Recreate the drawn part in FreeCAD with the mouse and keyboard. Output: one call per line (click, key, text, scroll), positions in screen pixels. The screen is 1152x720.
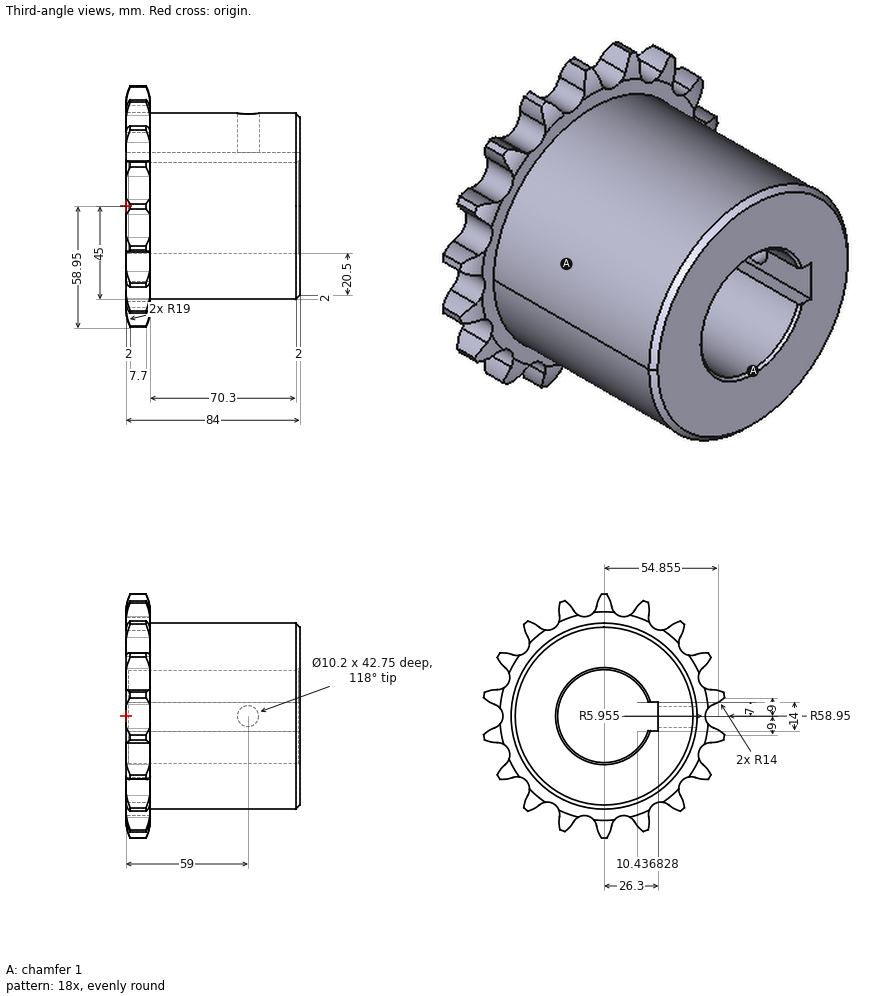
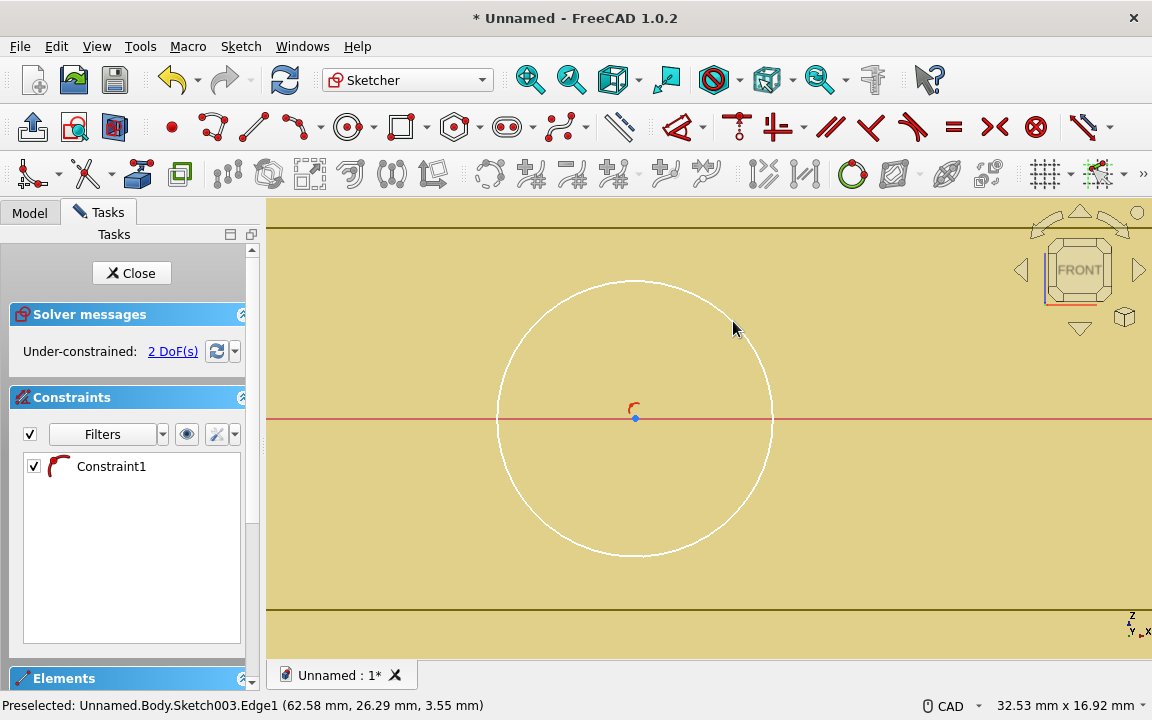
click(676, 128)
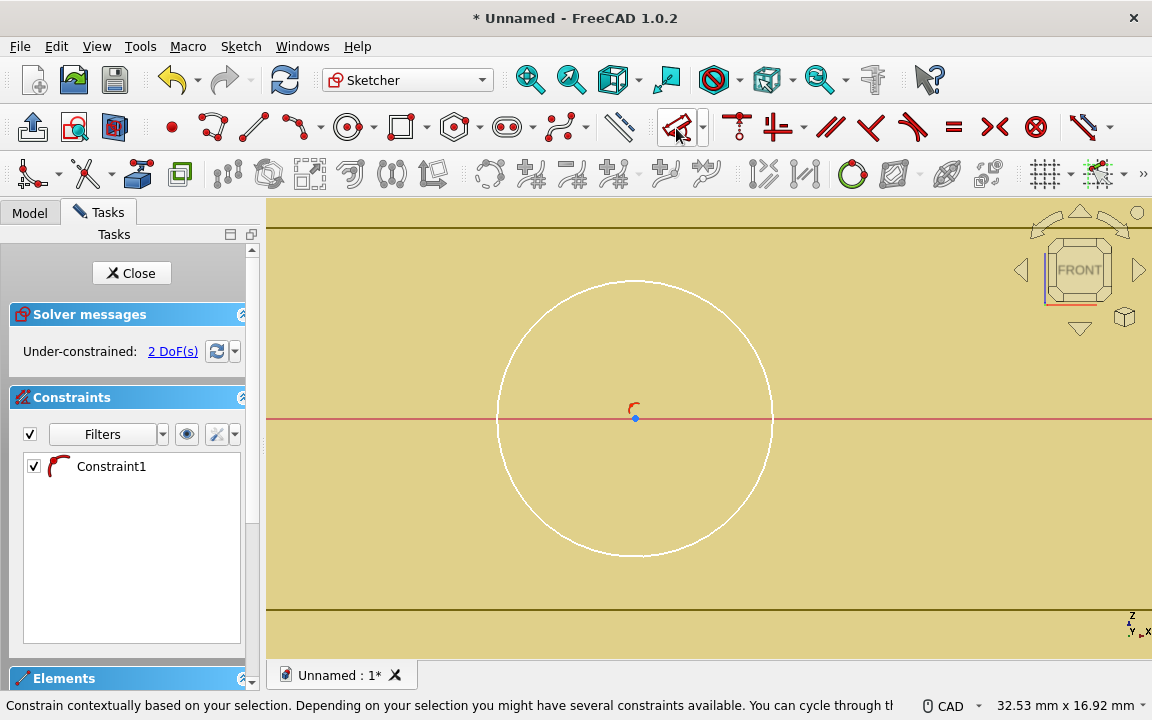
click(732, 321)
click(755, 298)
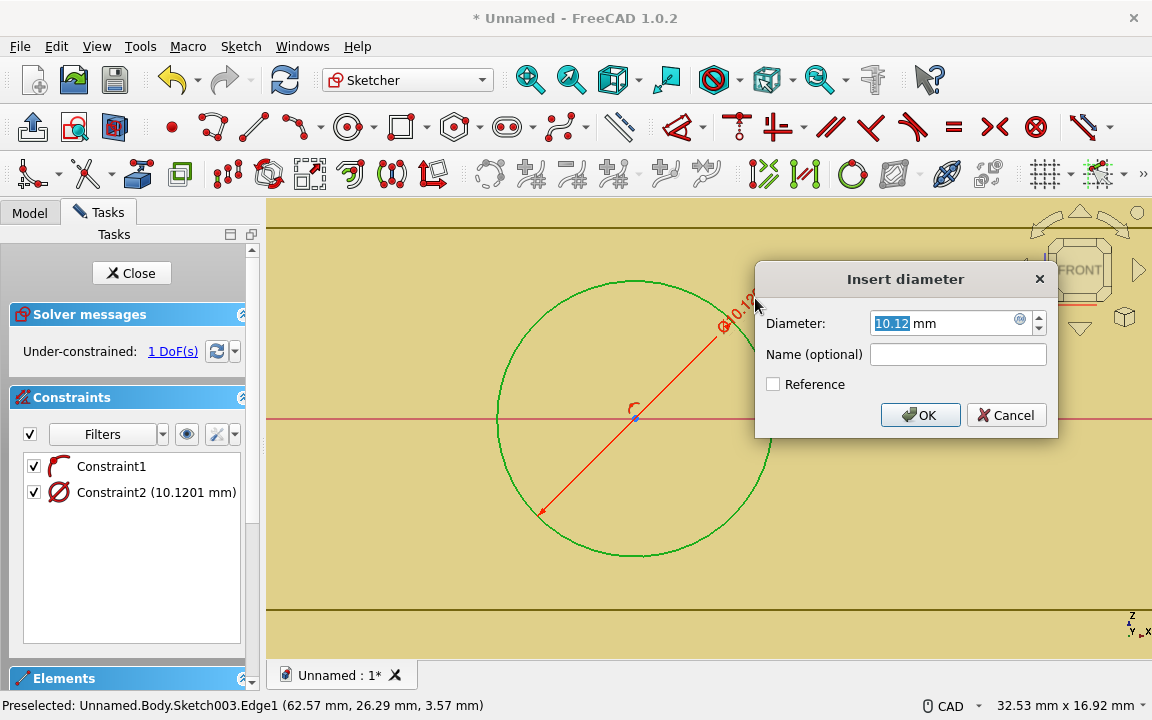
text(10.2)
key(Return)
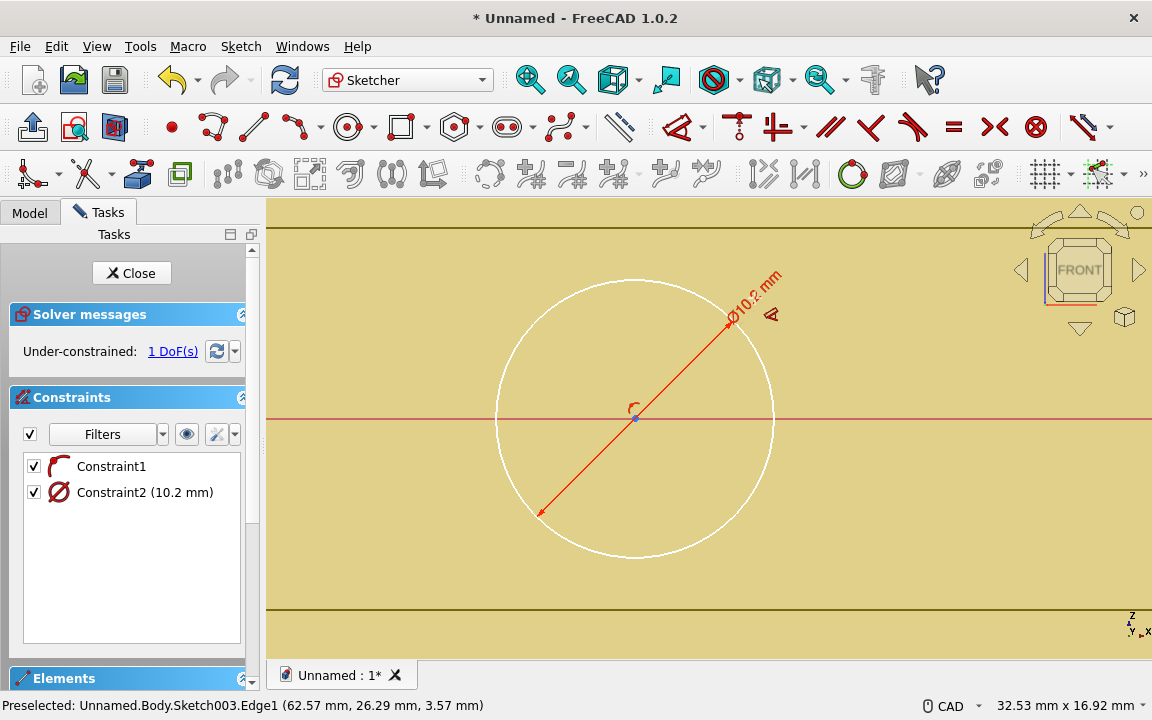
click(635, 419)
click(464, 453)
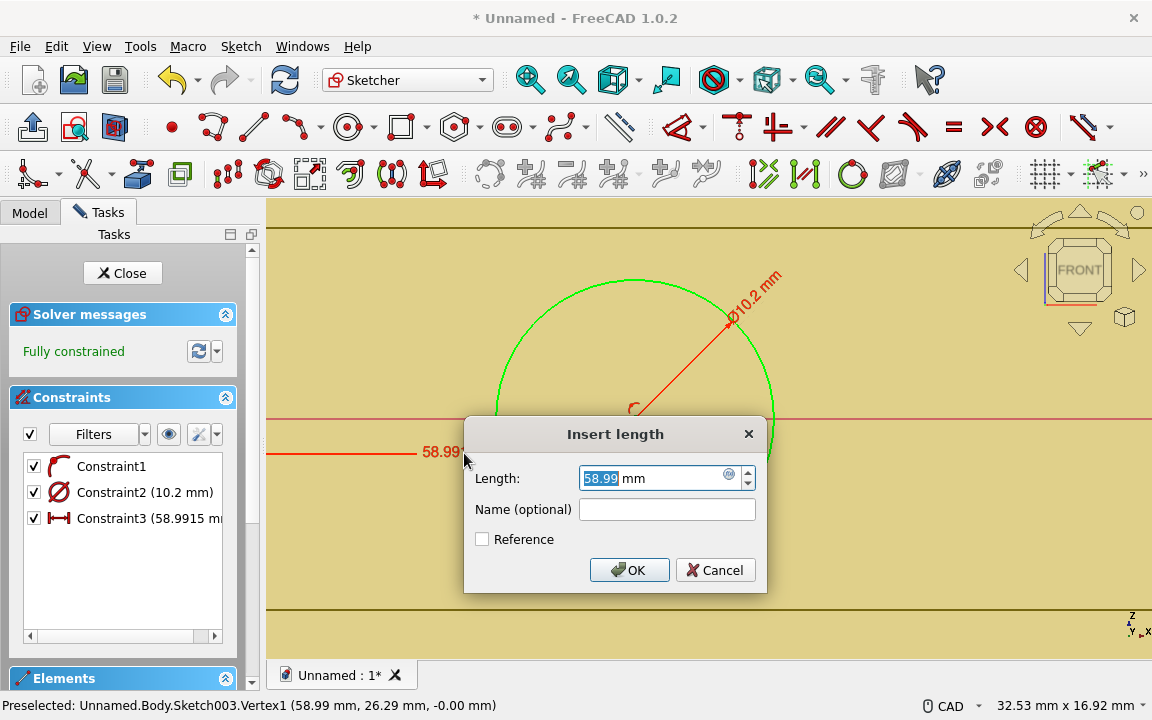
text(59)
key(Return)
key(Escape)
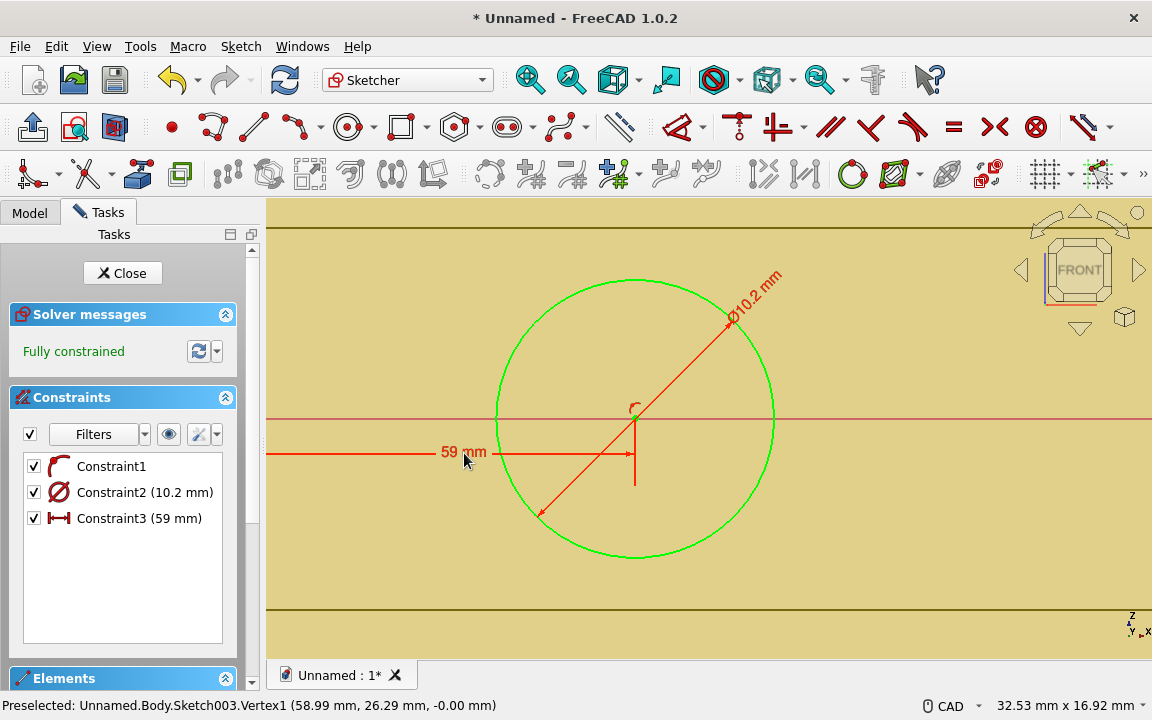
click(123, 273)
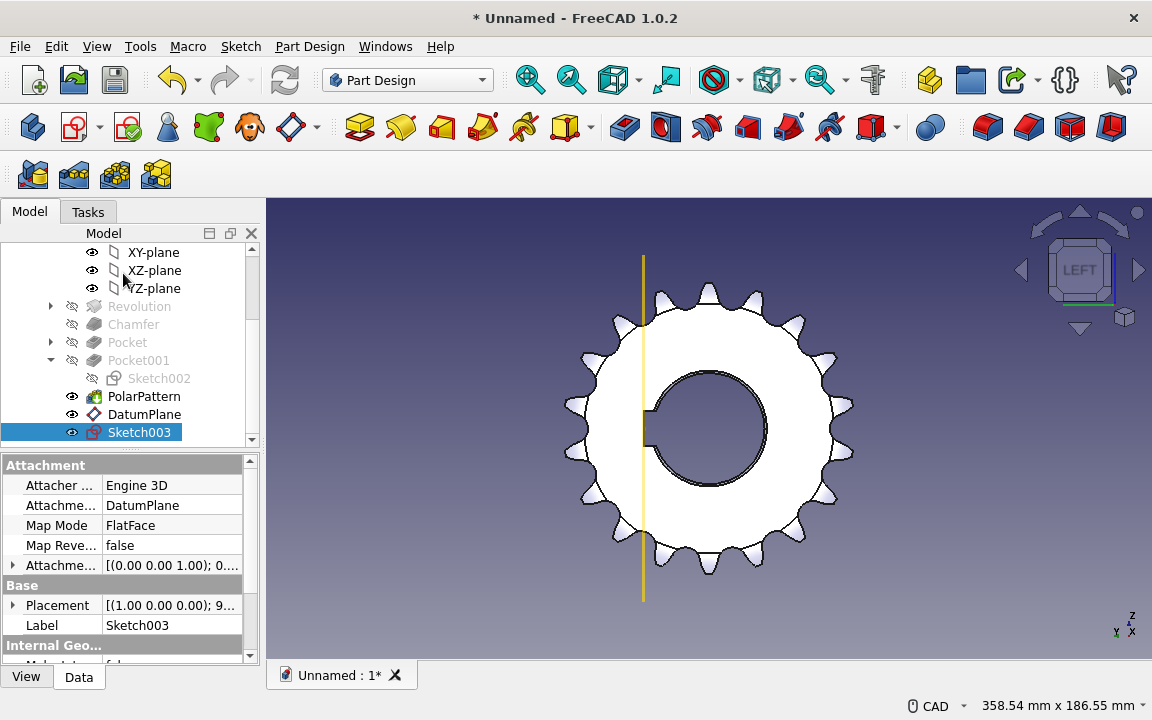
click(666, 128)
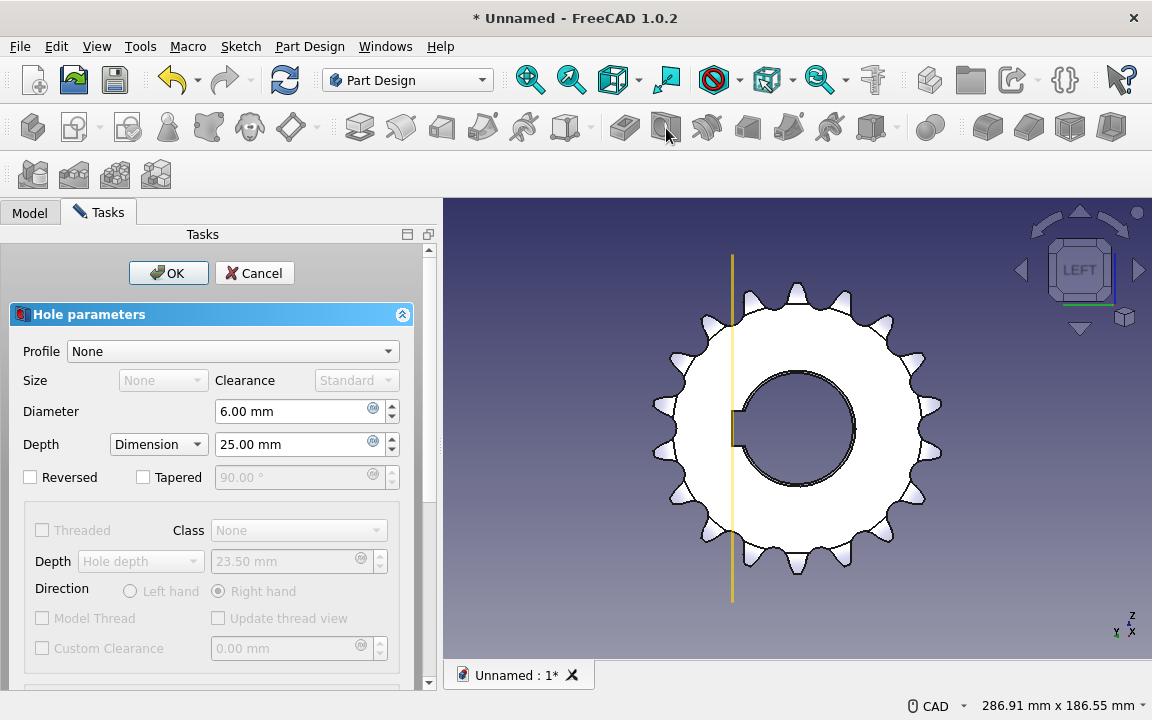
triple_click(300, 412)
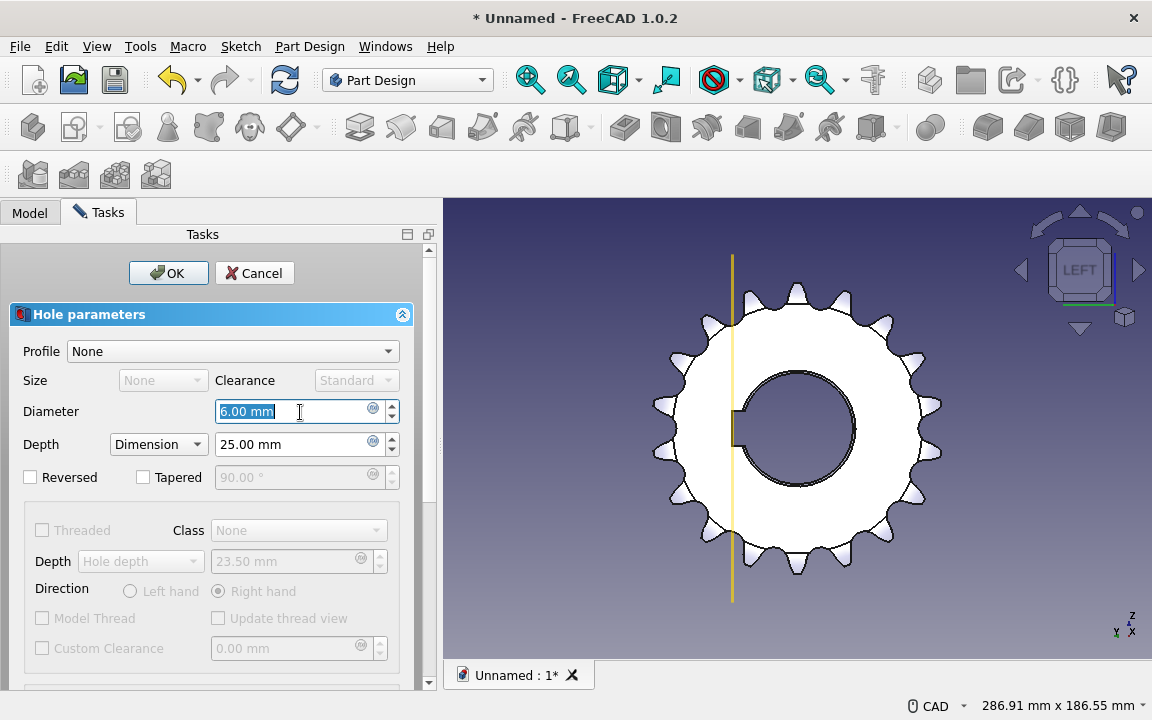
text(10.2)
key(Tab)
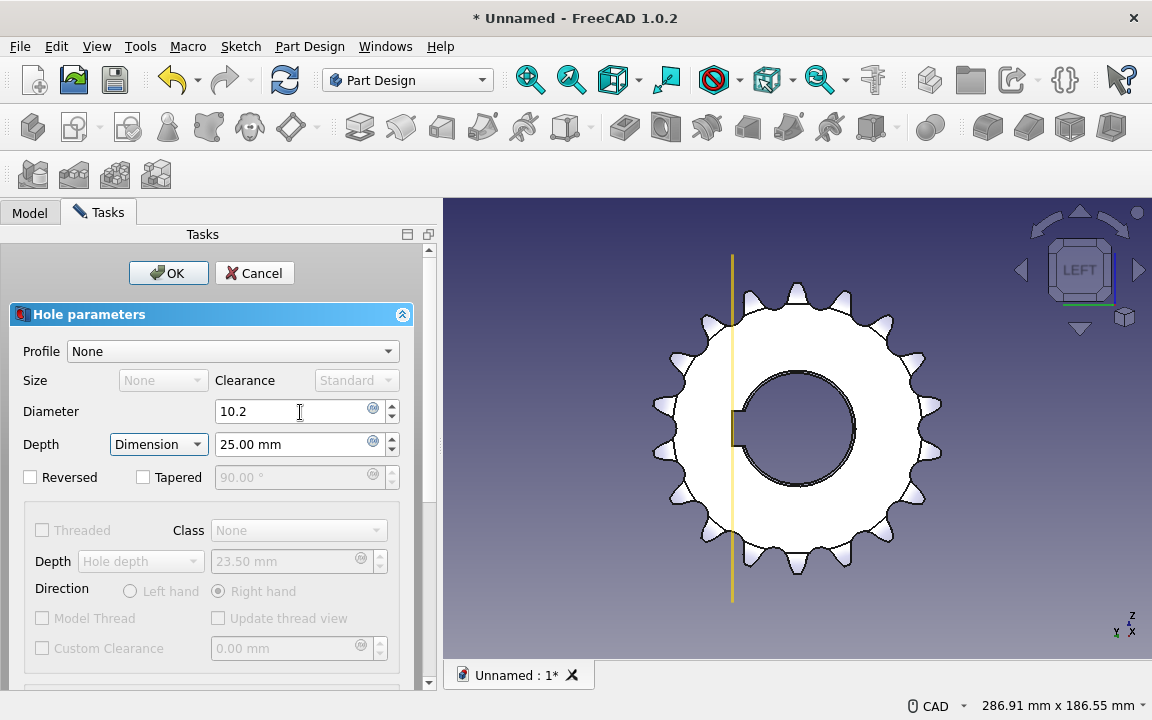
triple_click(300, 444)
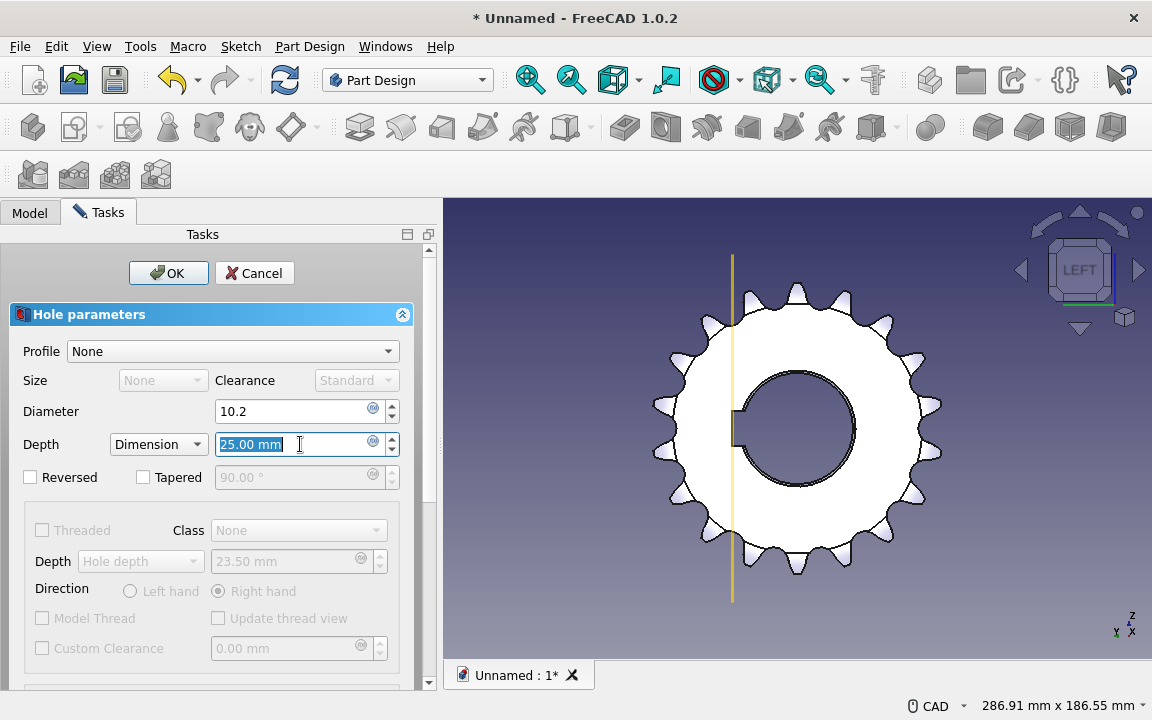
text(42.75)
key(Tab)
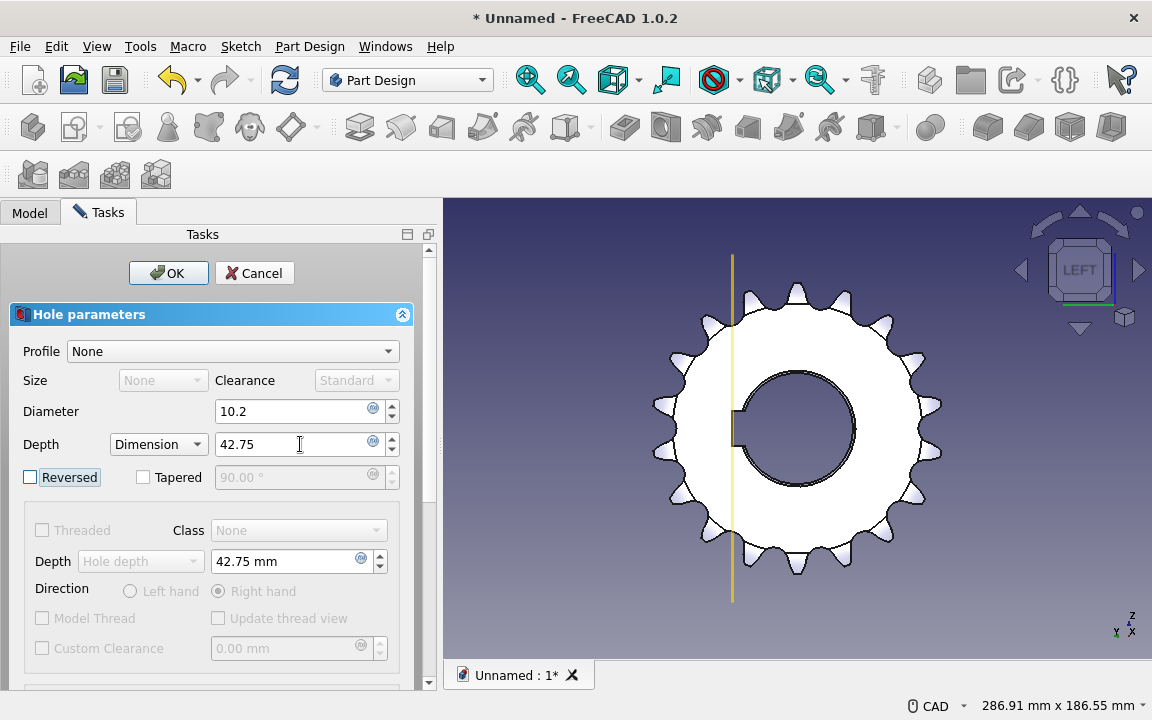
click(169, 273)